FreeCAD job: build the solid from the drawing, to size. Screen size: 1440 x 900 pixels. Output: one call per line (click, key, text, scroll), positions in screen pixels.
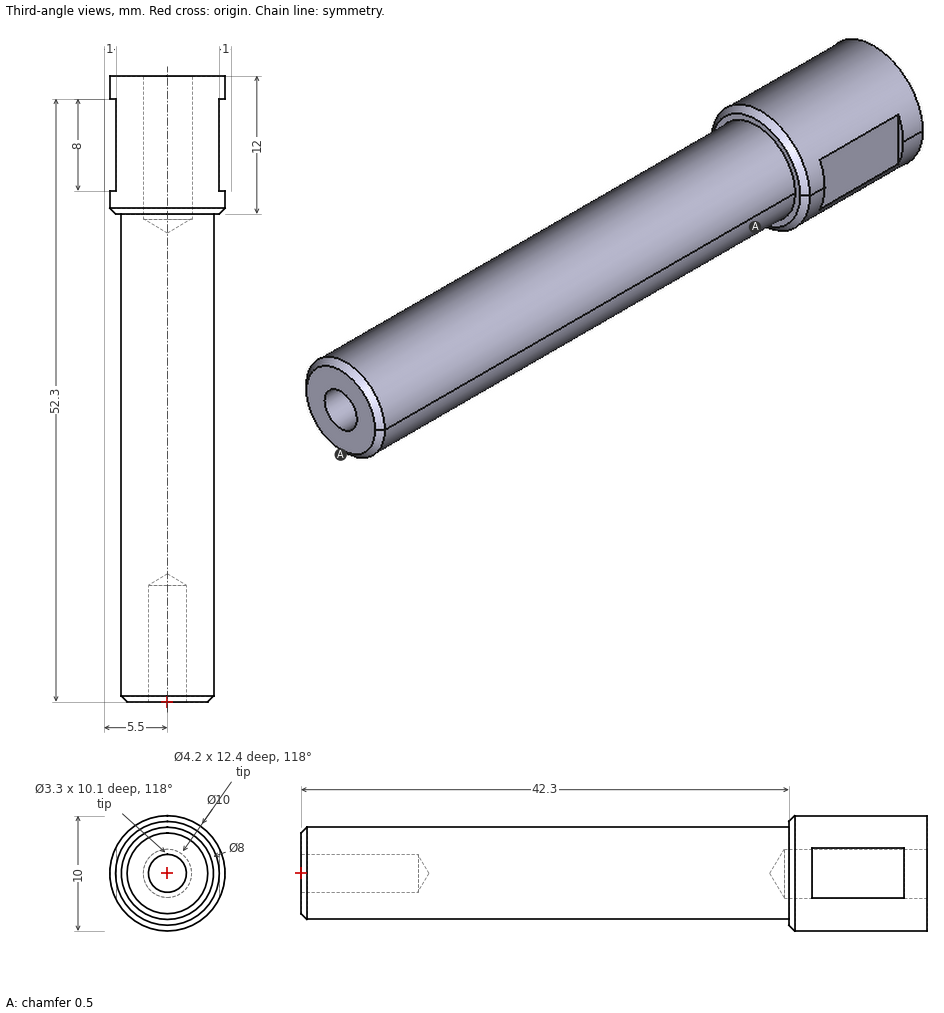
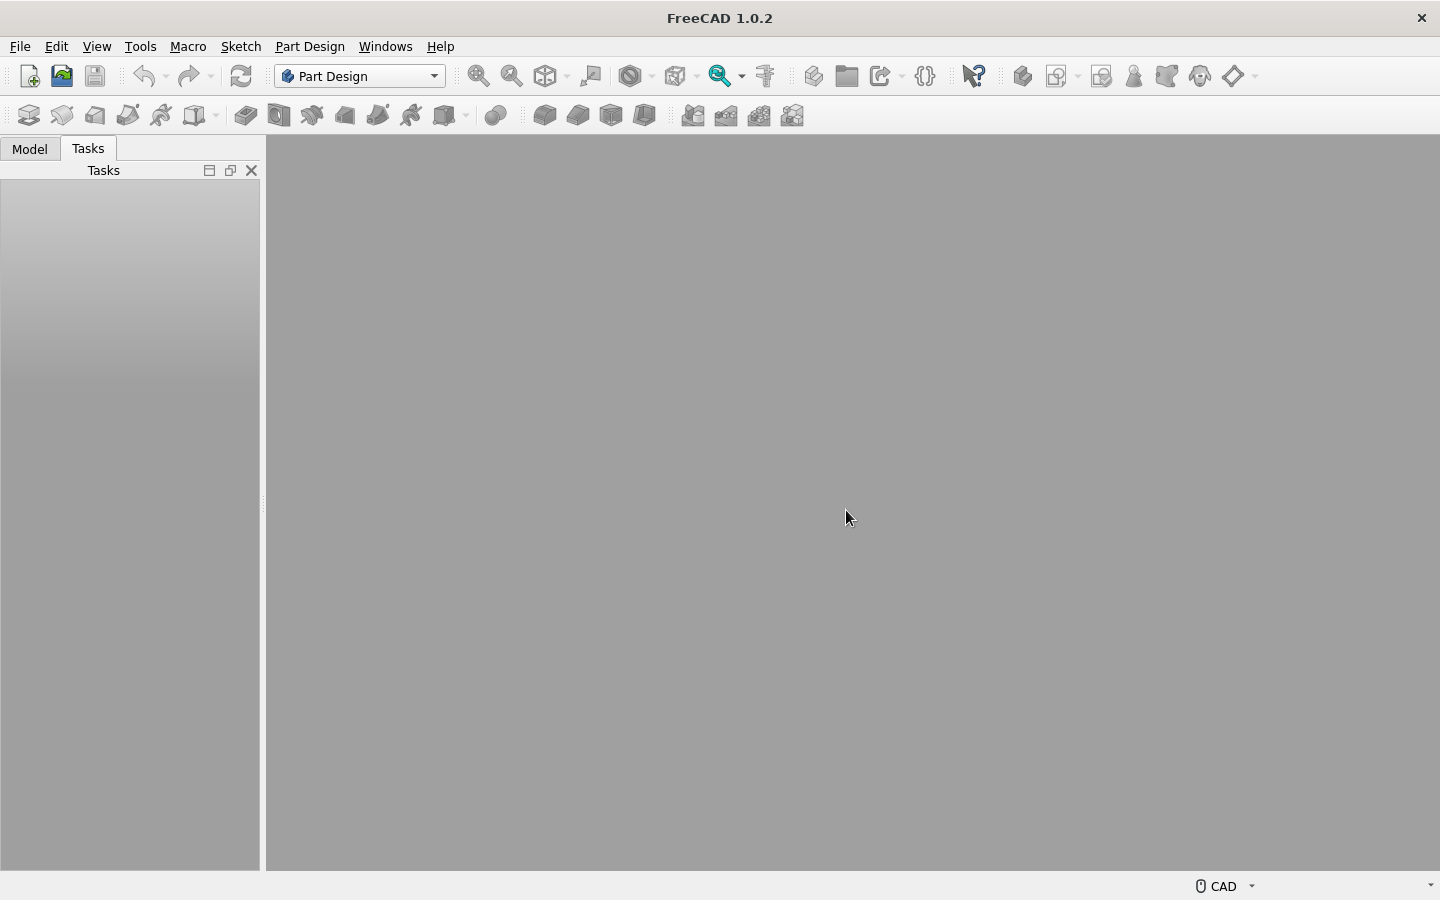
key(ctrl+n)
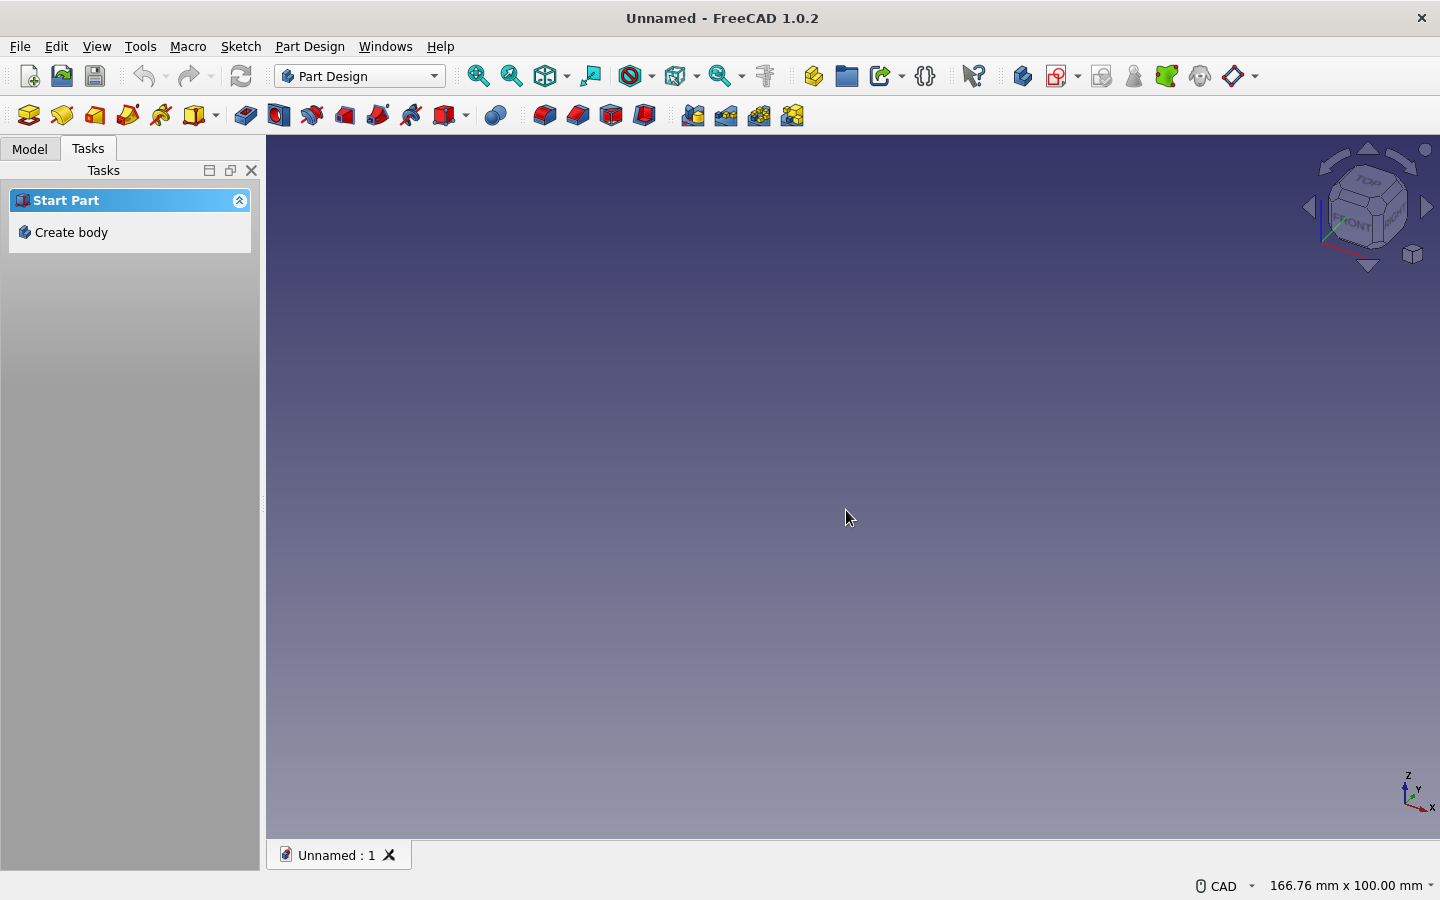
click(1056, 76)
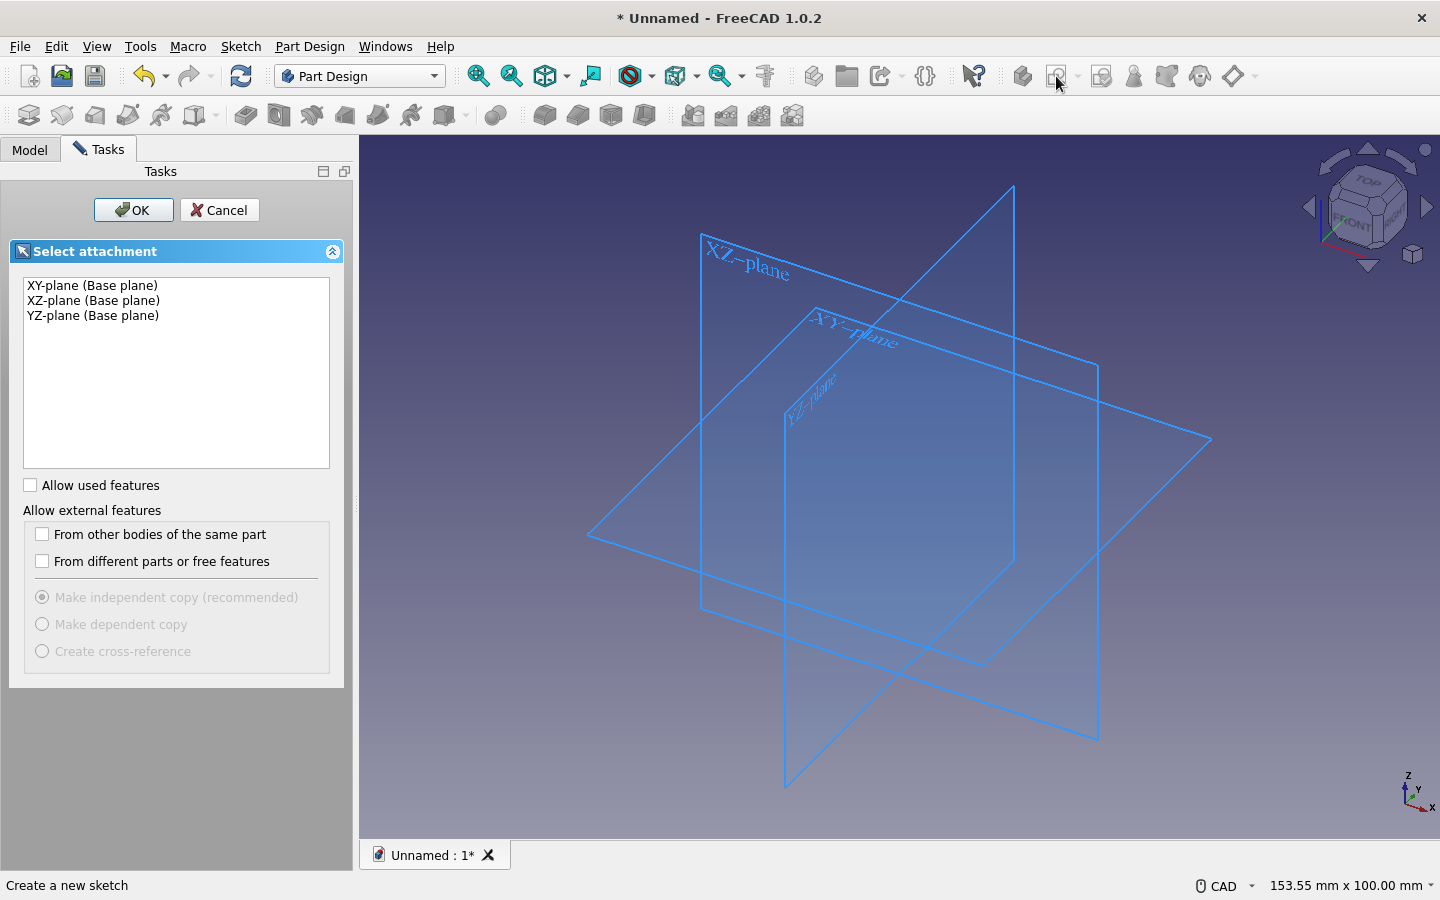
click(84, 300)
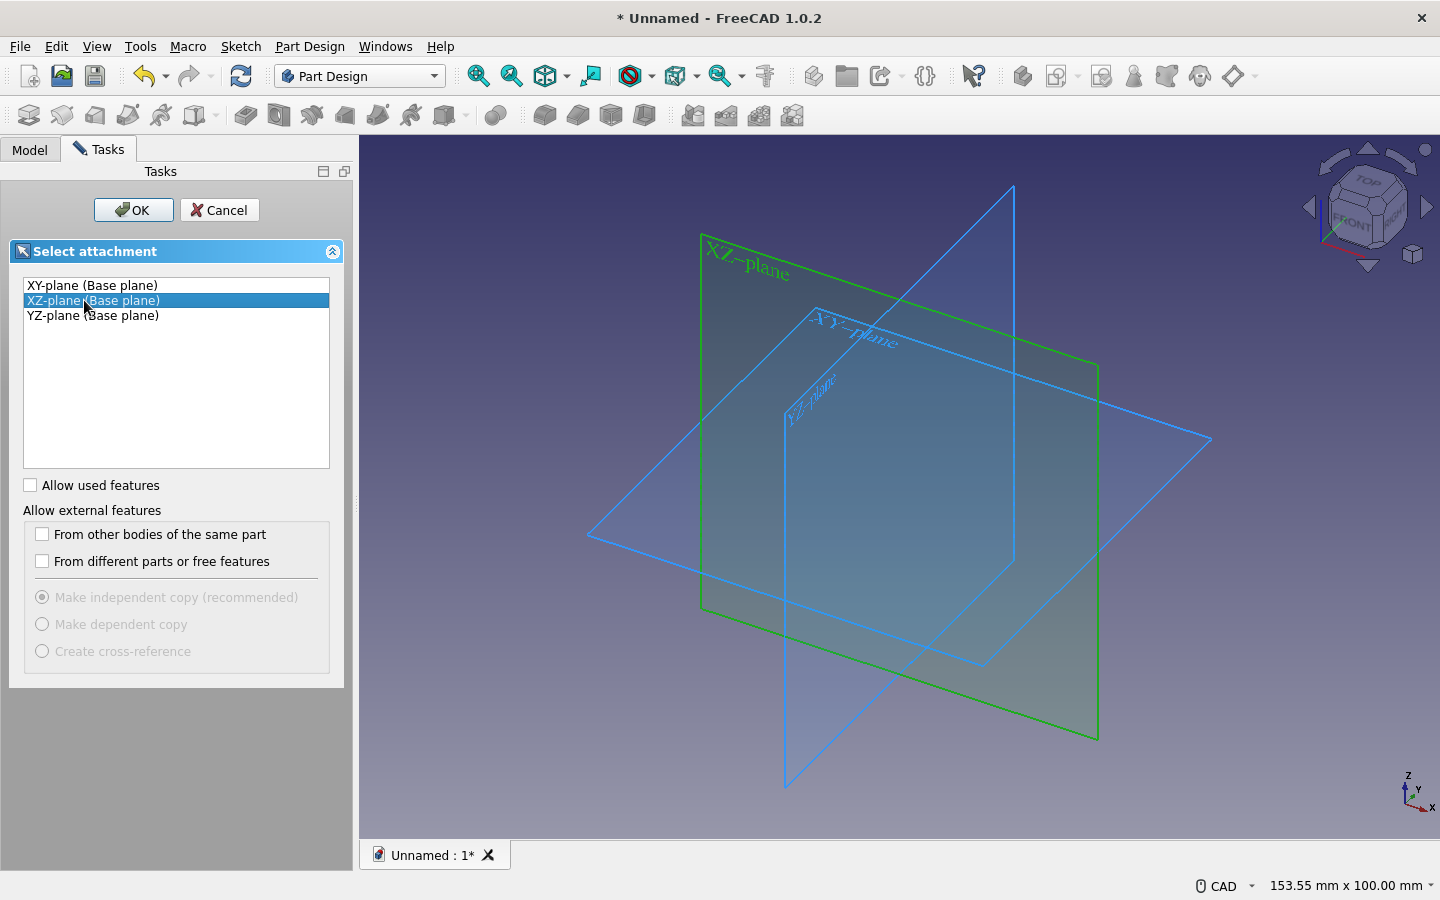
click(134, 210)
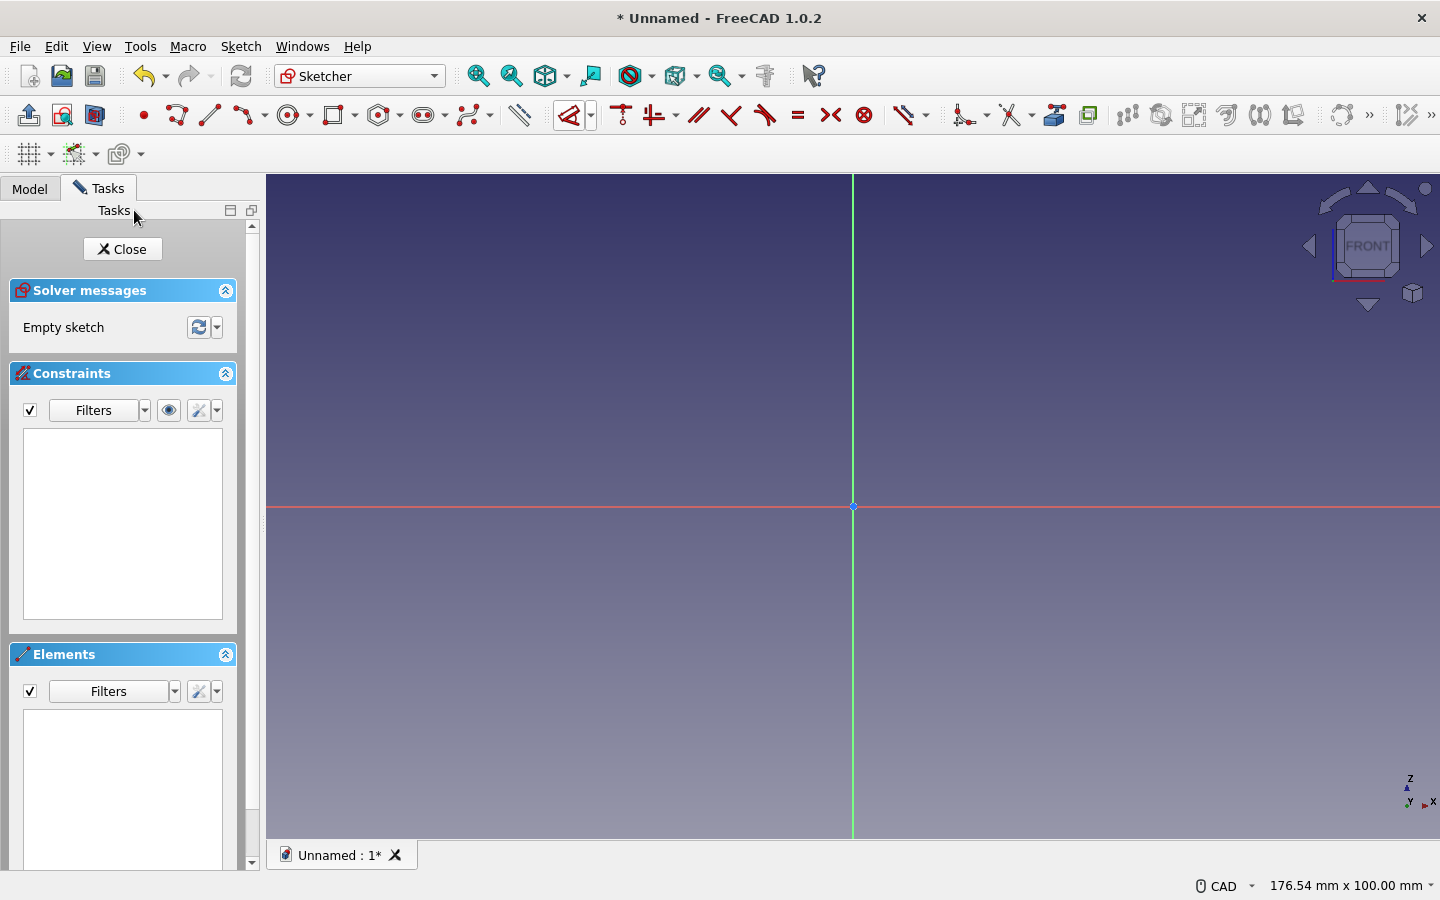
scroll(864, 506, up, 10)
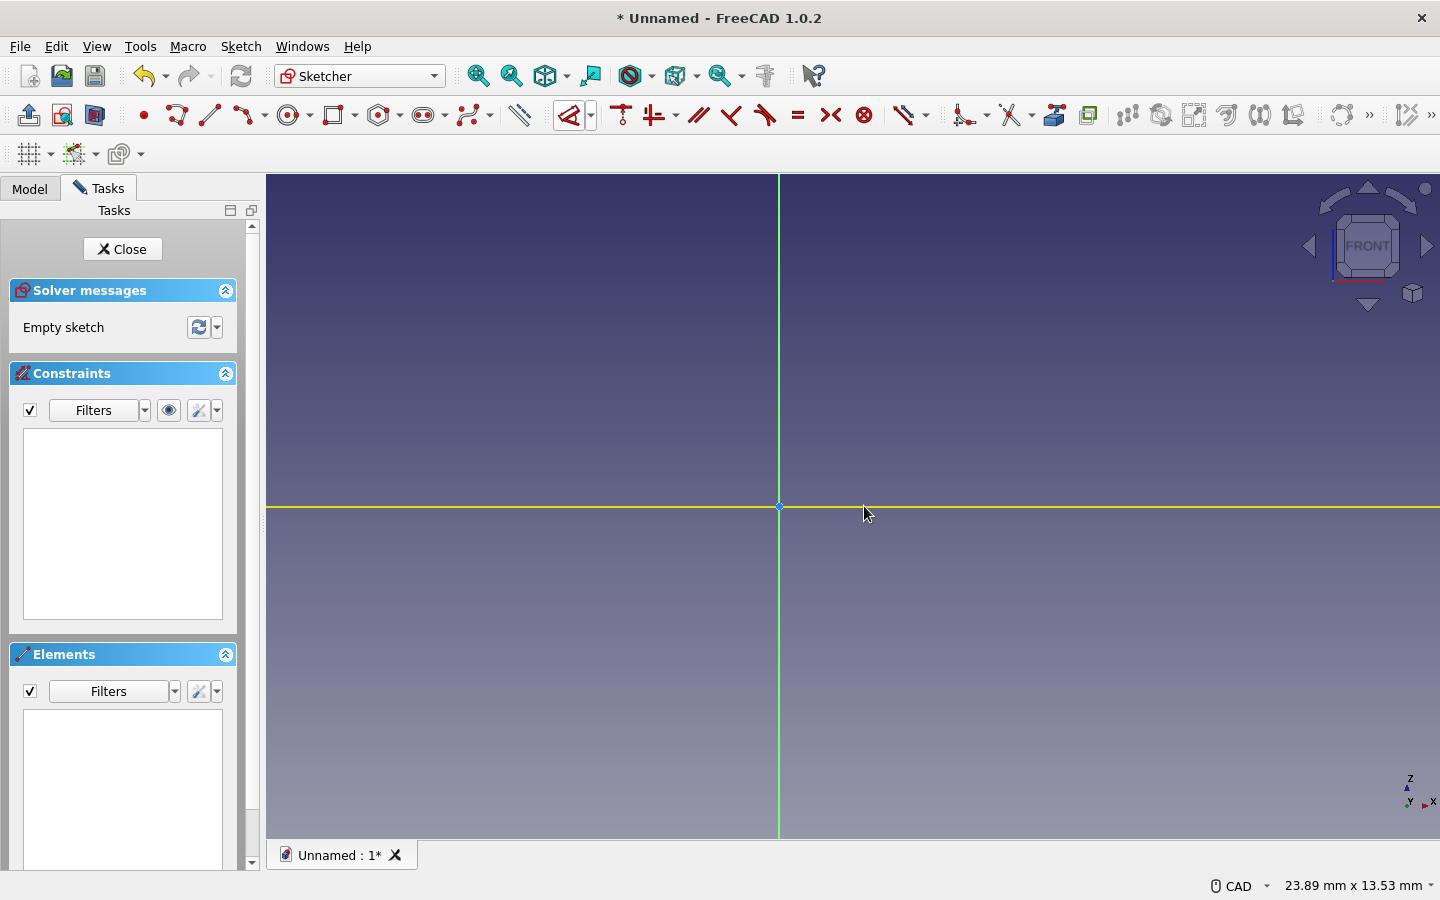
key(g)
key(c)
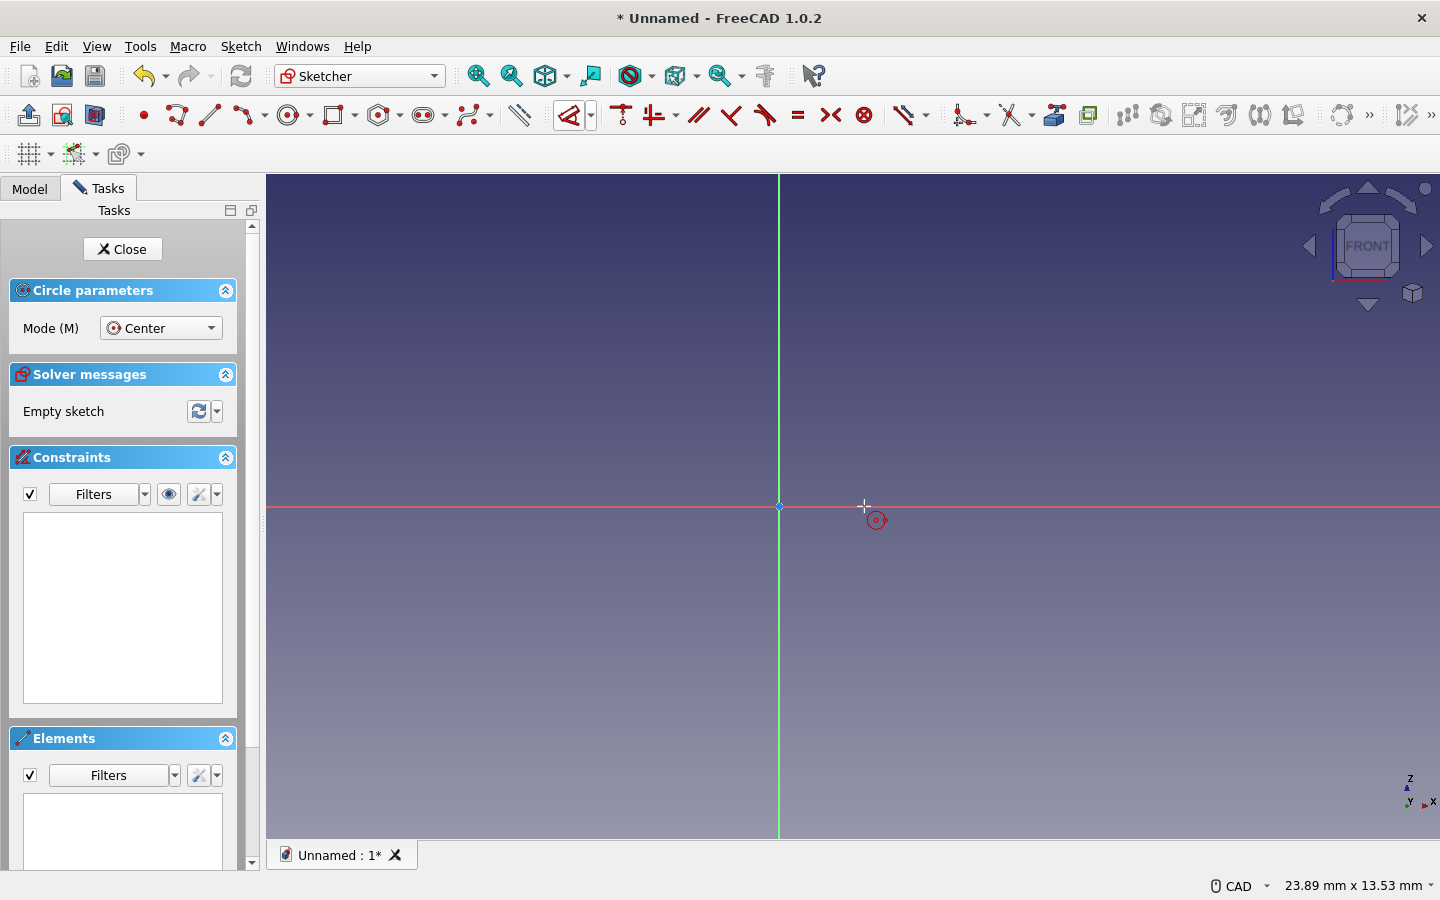
click(779, 506)
move(918, 368)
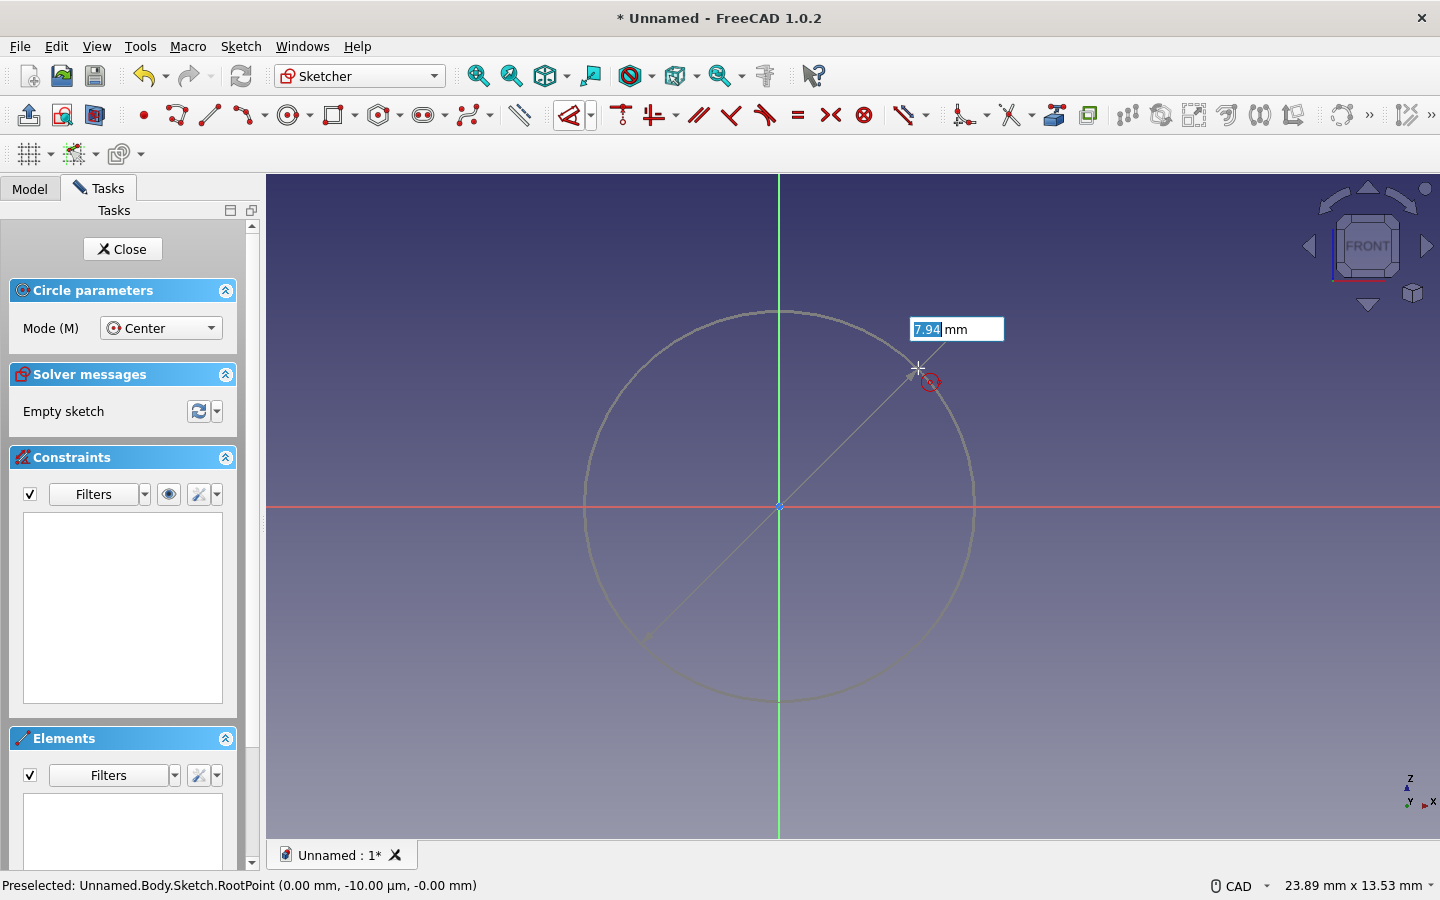
text(8)
key(Return)
key(Escape)